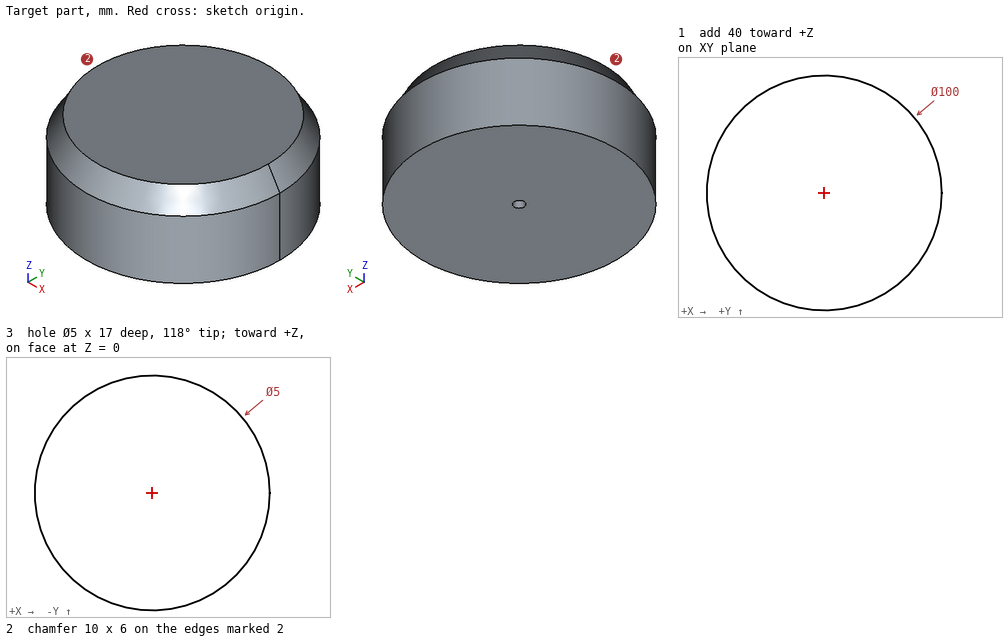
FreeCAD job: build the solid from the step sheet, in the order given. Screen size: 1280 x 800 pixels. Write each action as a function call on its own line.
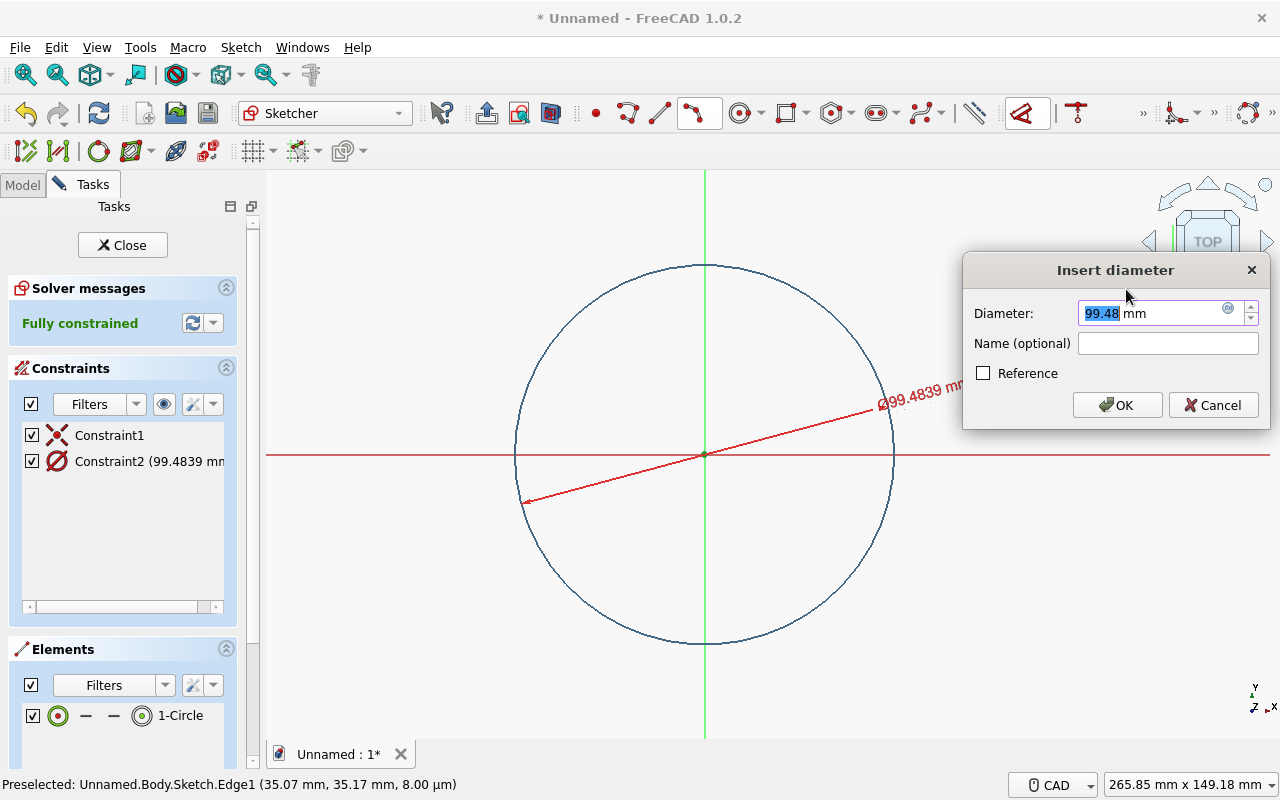
text(100)
key(Return)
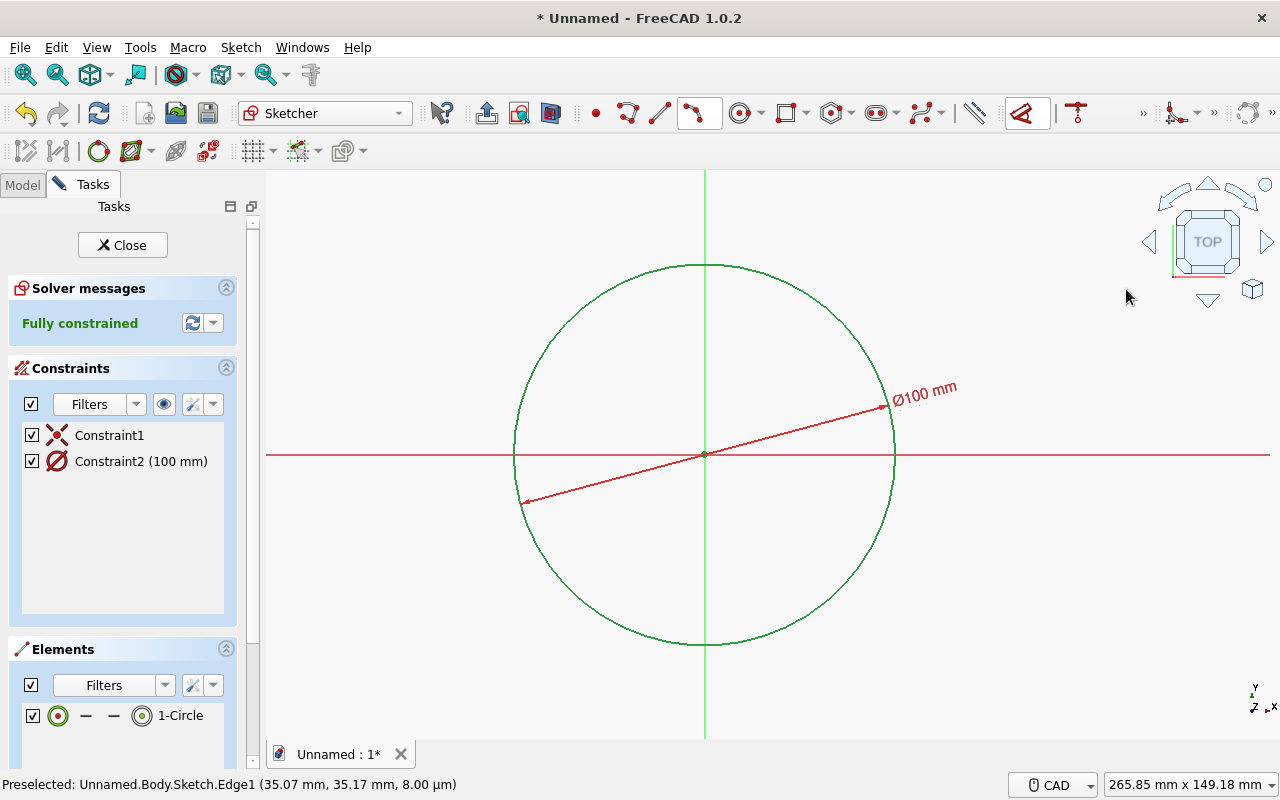
click(123, 245)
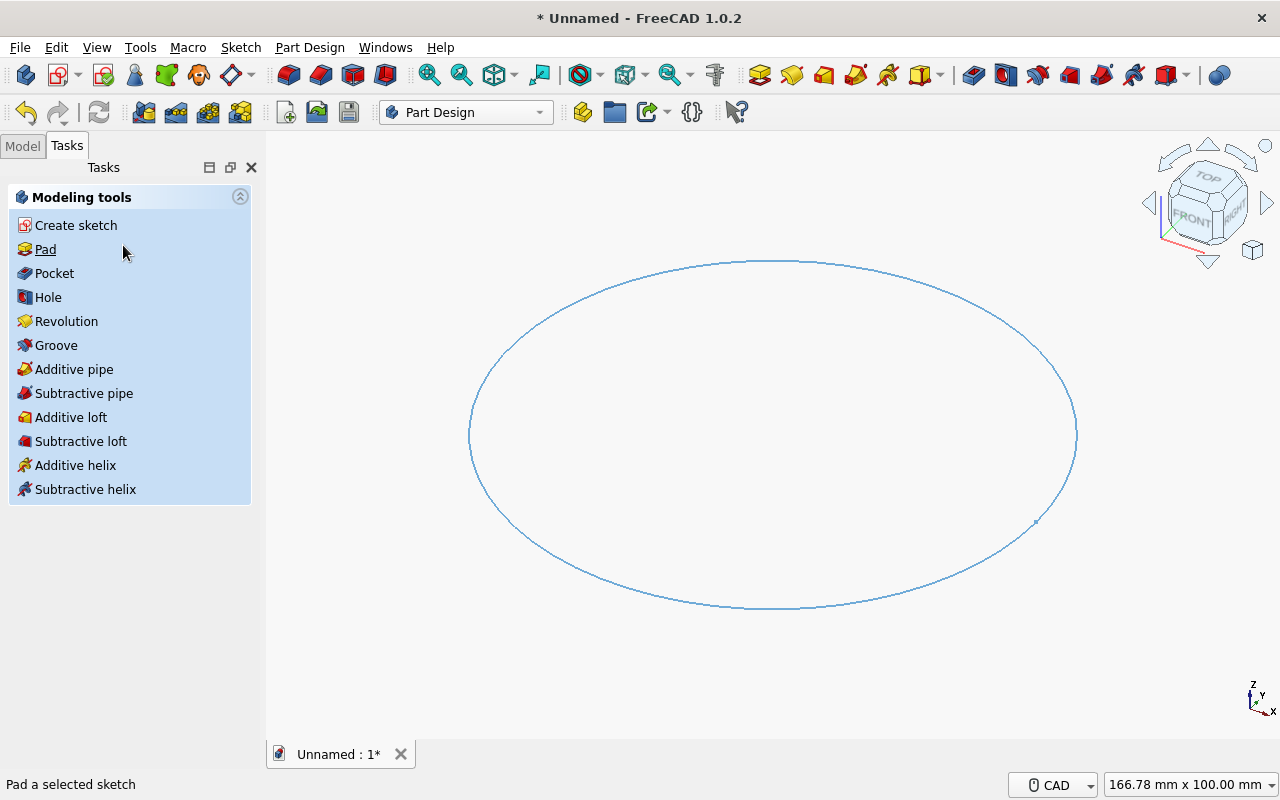
click(760, 76)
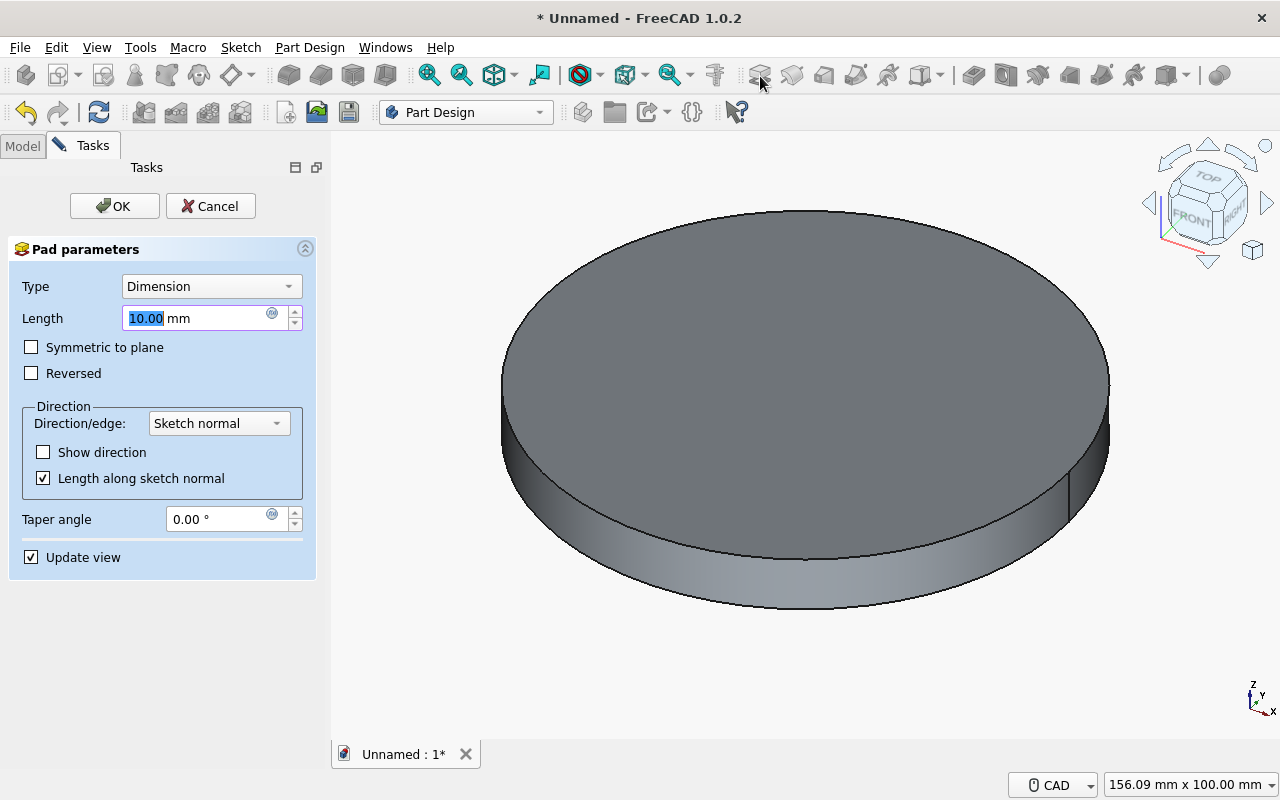
text(40)
key(Tab)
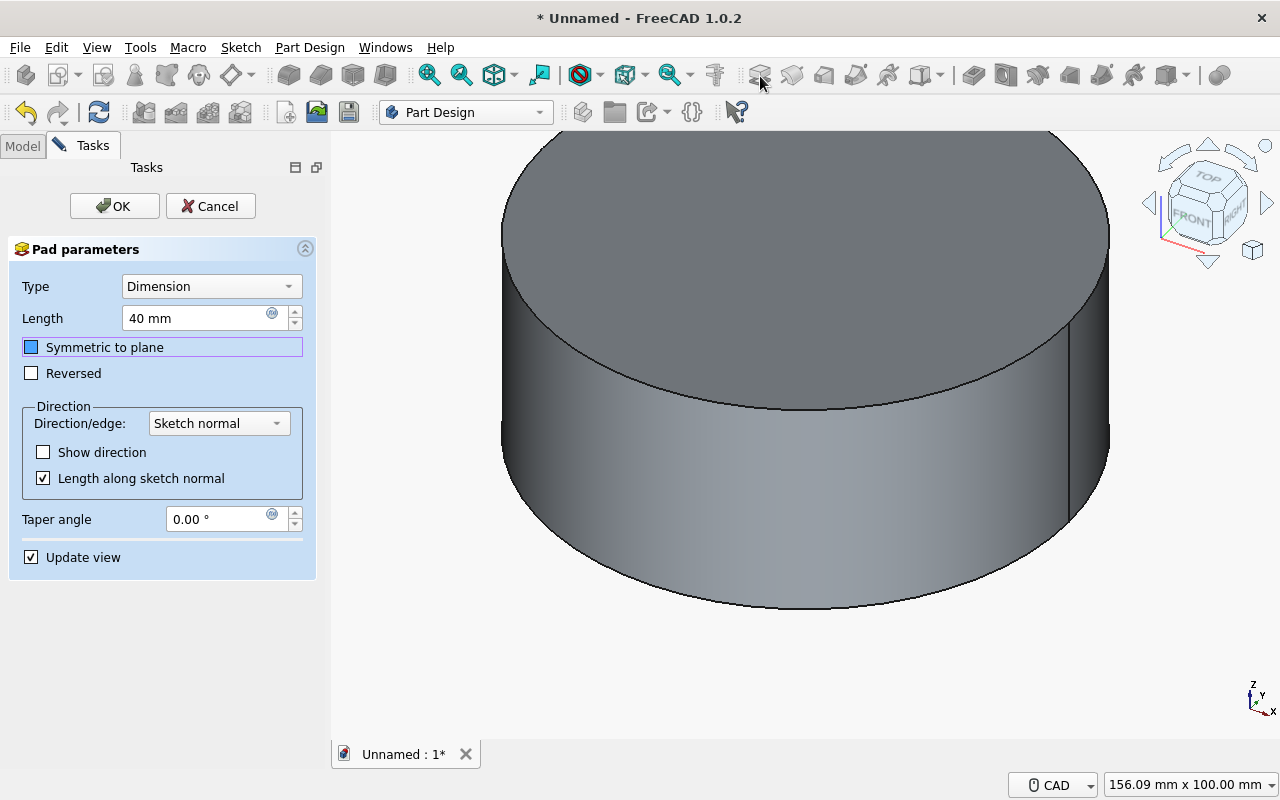
click(115, 206)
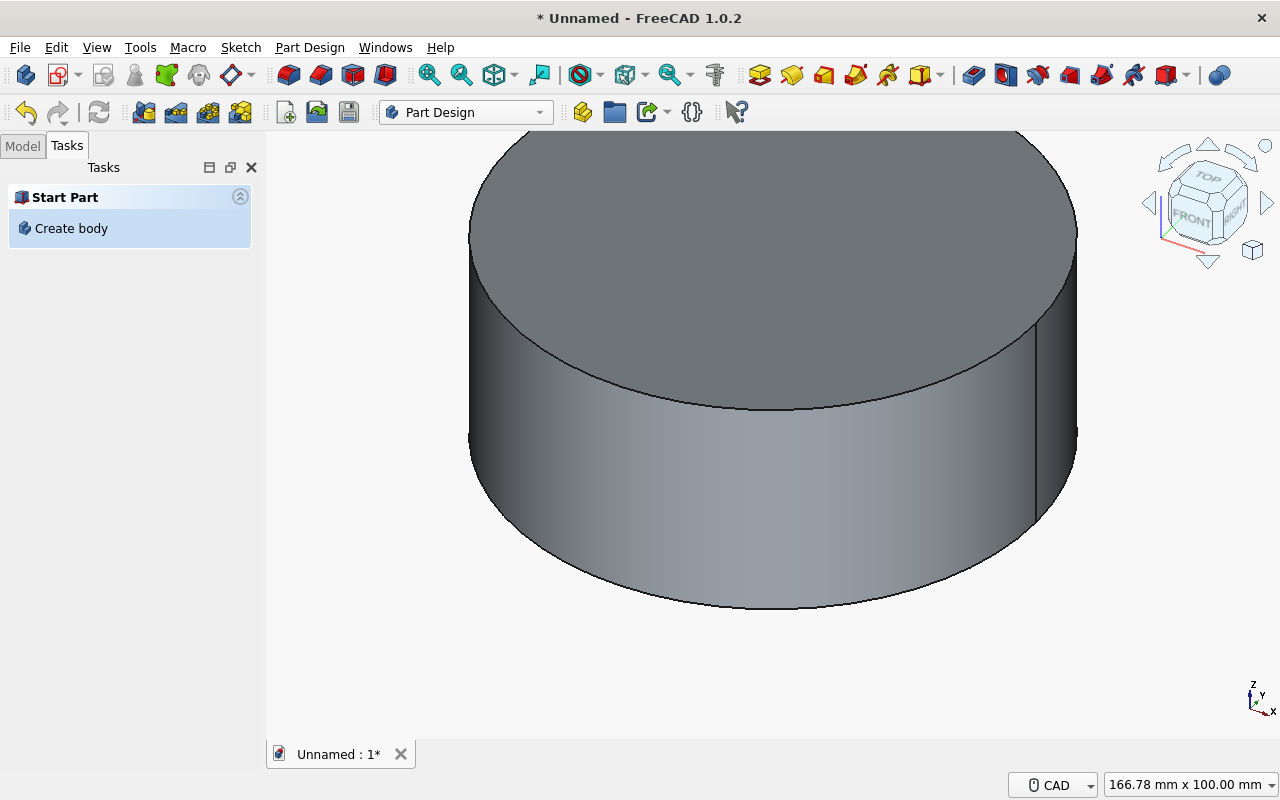
click(430, 76)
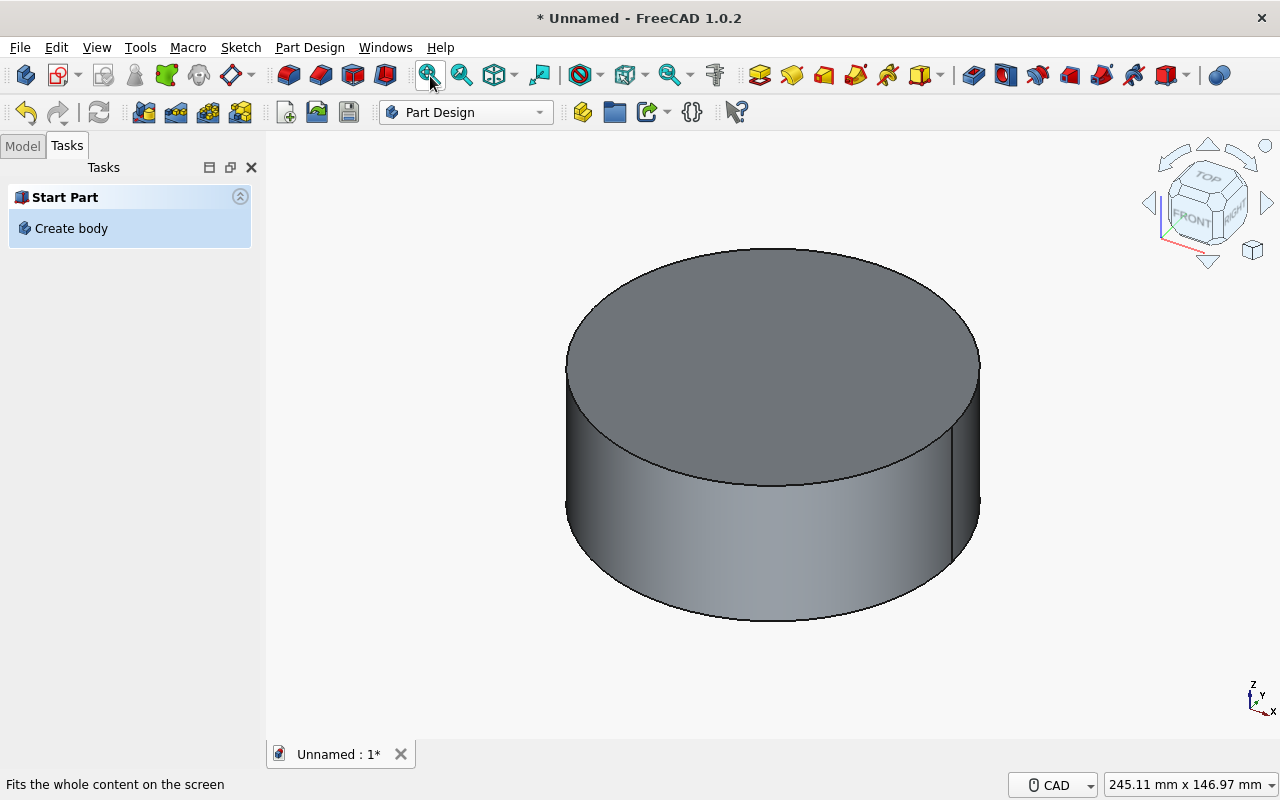
click(567, 379)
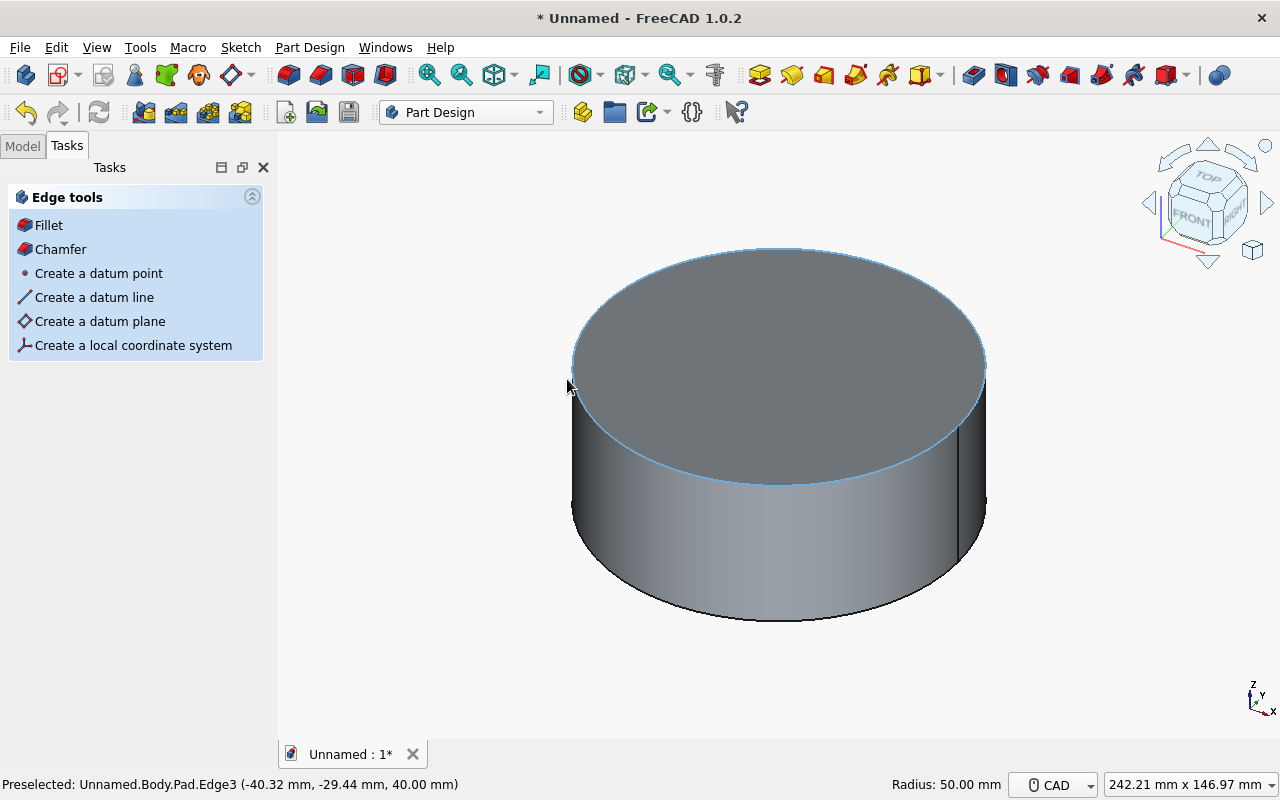
click(322, 76)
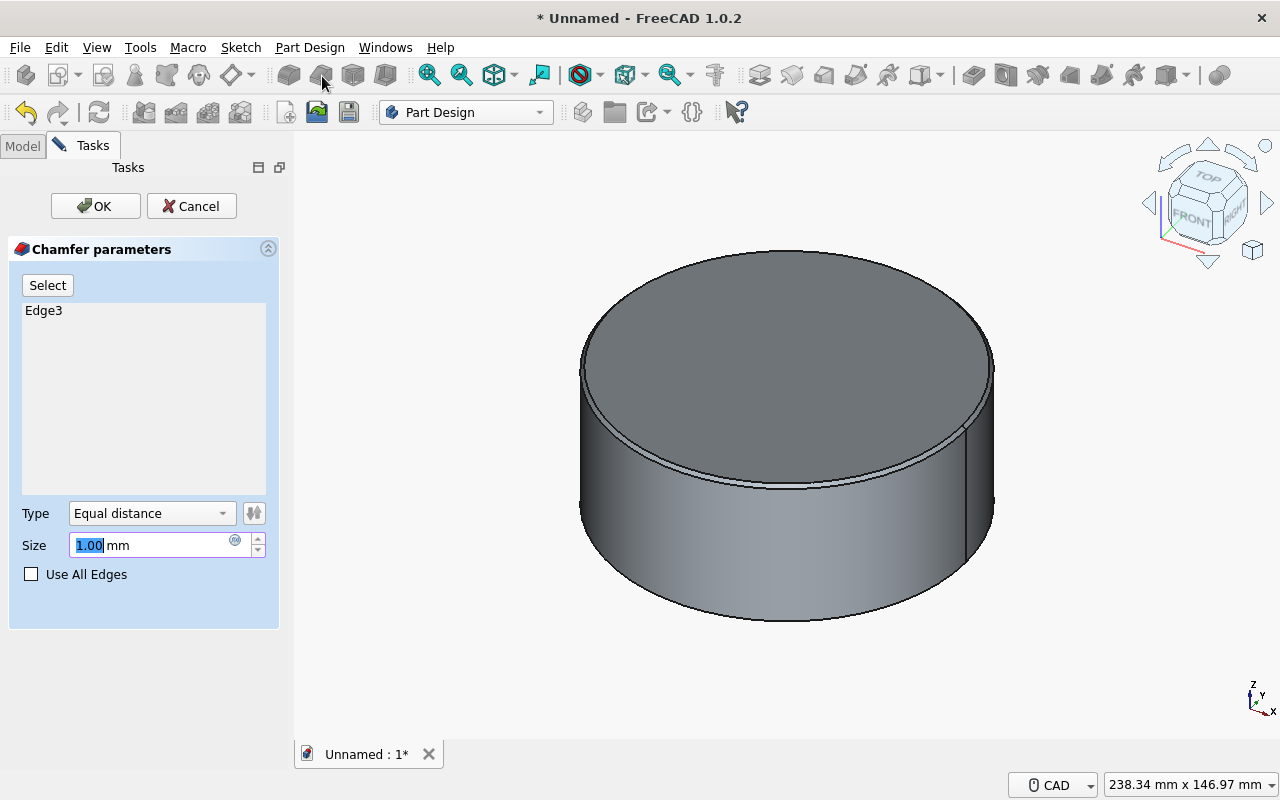
text(10)
key(Tab)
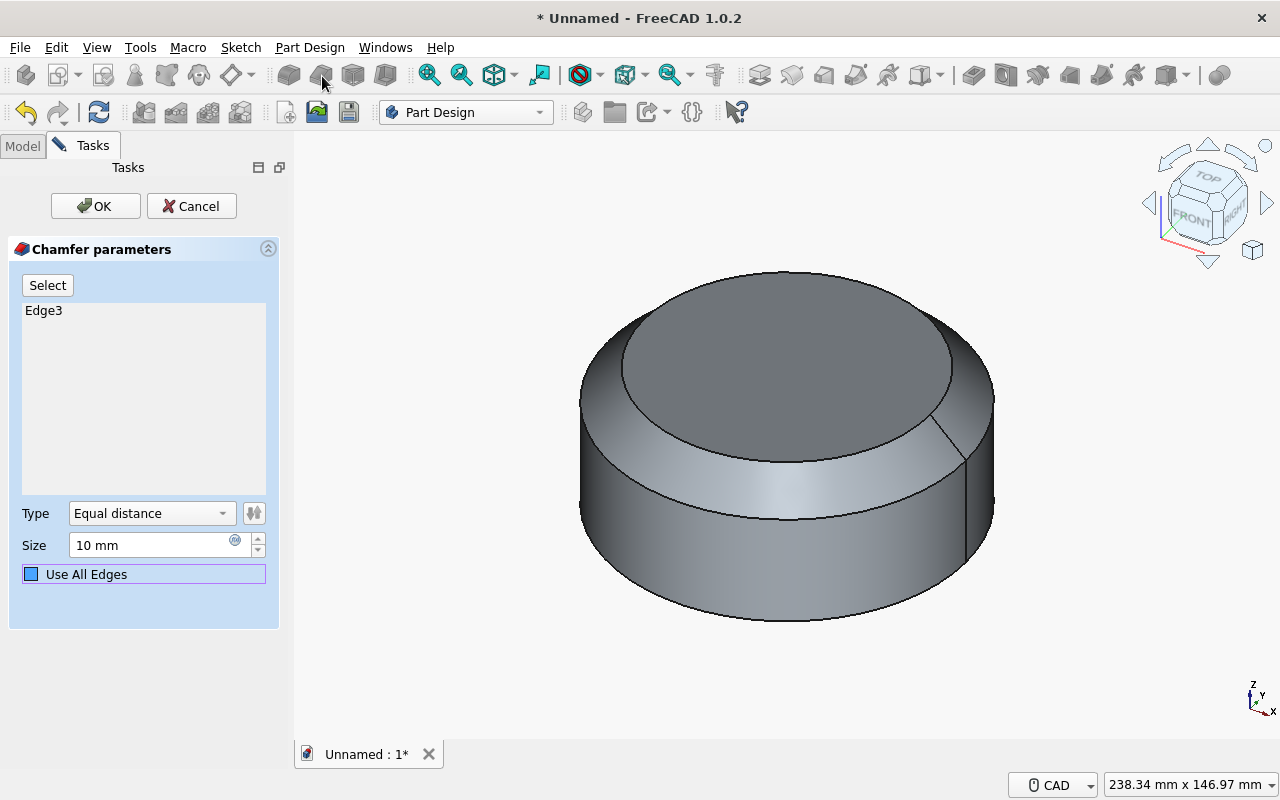
click(153, 514)